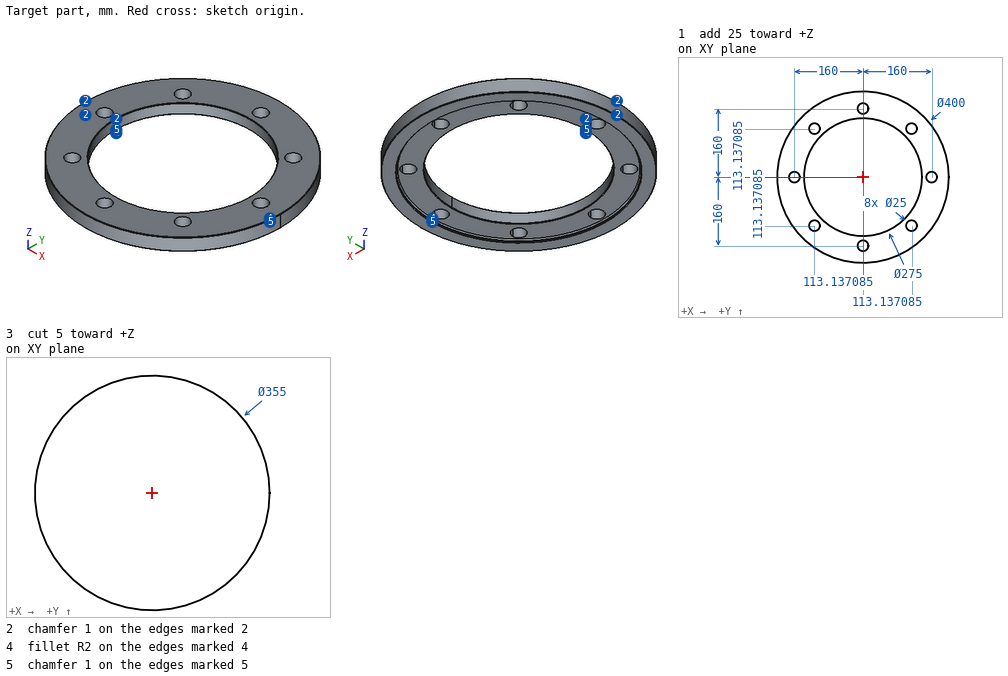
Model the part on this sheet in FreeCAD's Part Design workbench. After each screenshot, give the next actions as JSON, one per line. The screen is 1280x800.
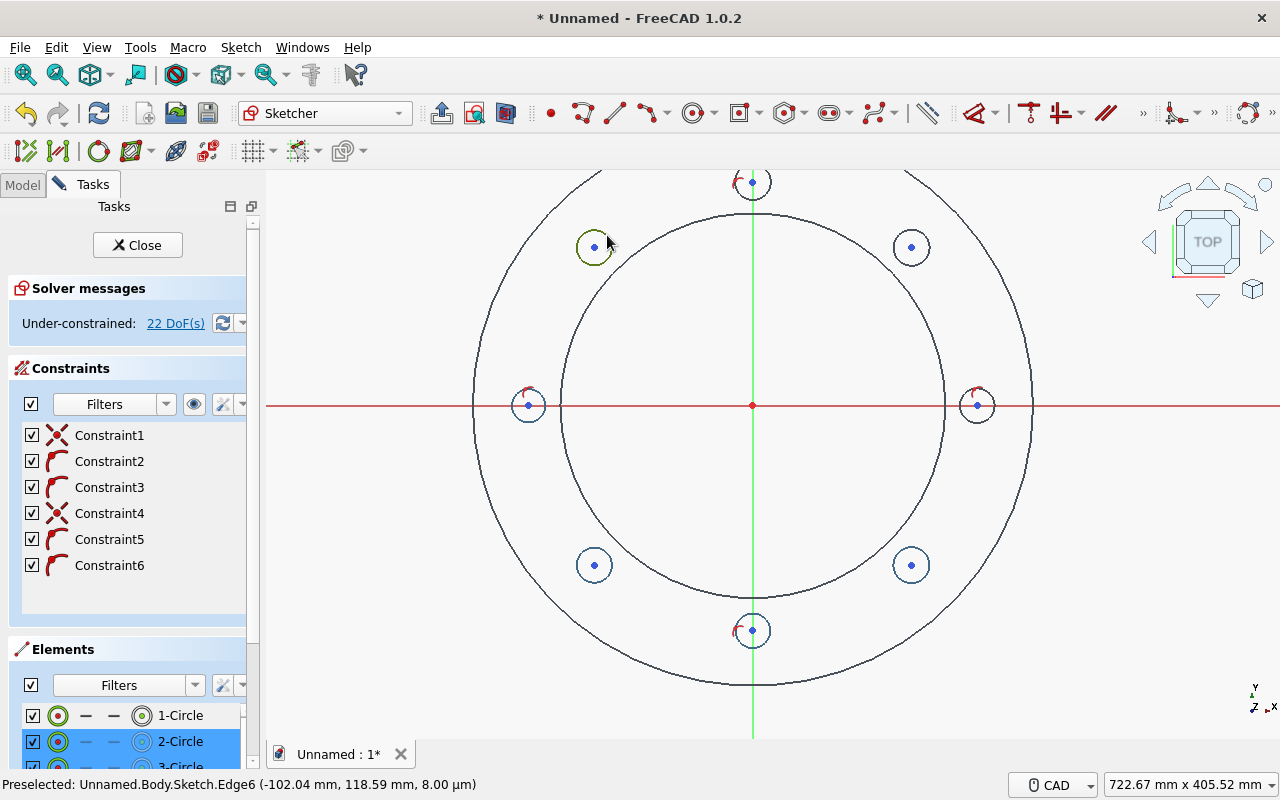
{"action": "left_click", "coordinate": [989, 393]}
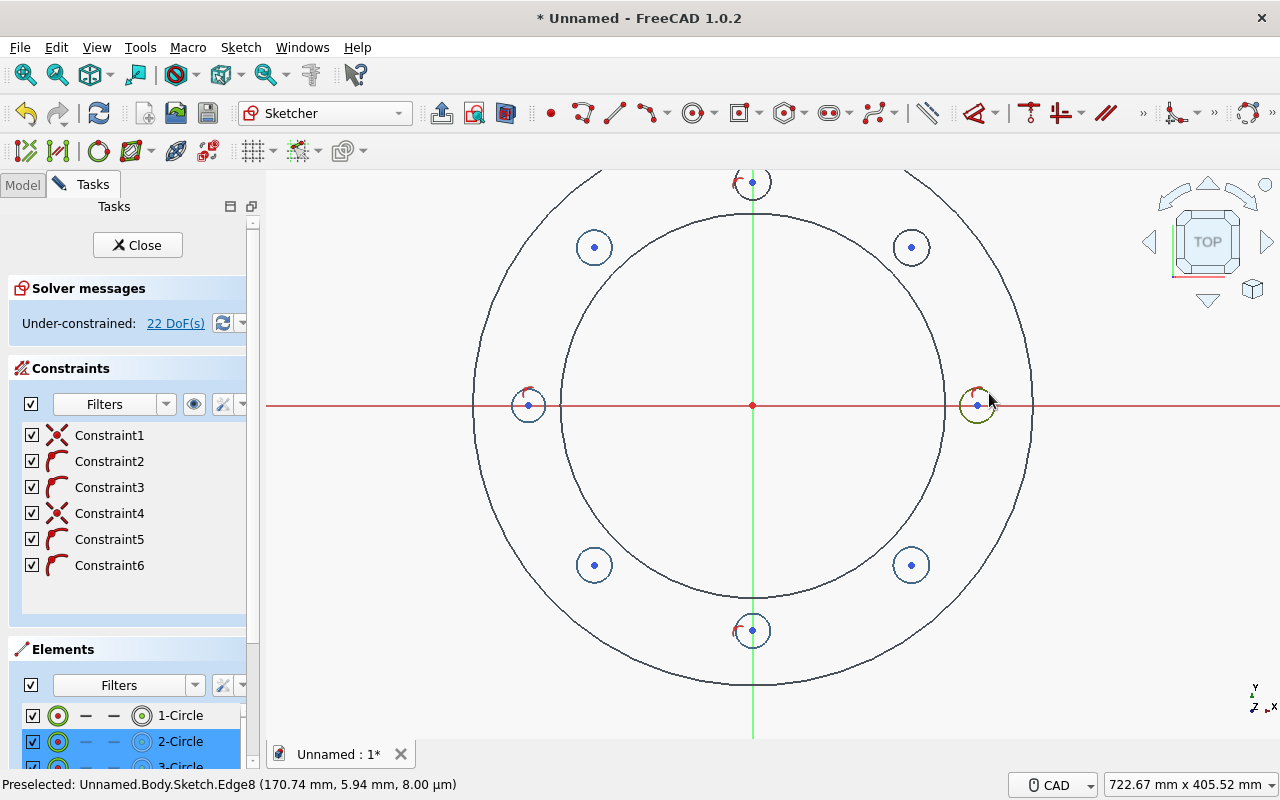
{"action": "left_click", "coordinate": [752, 200]}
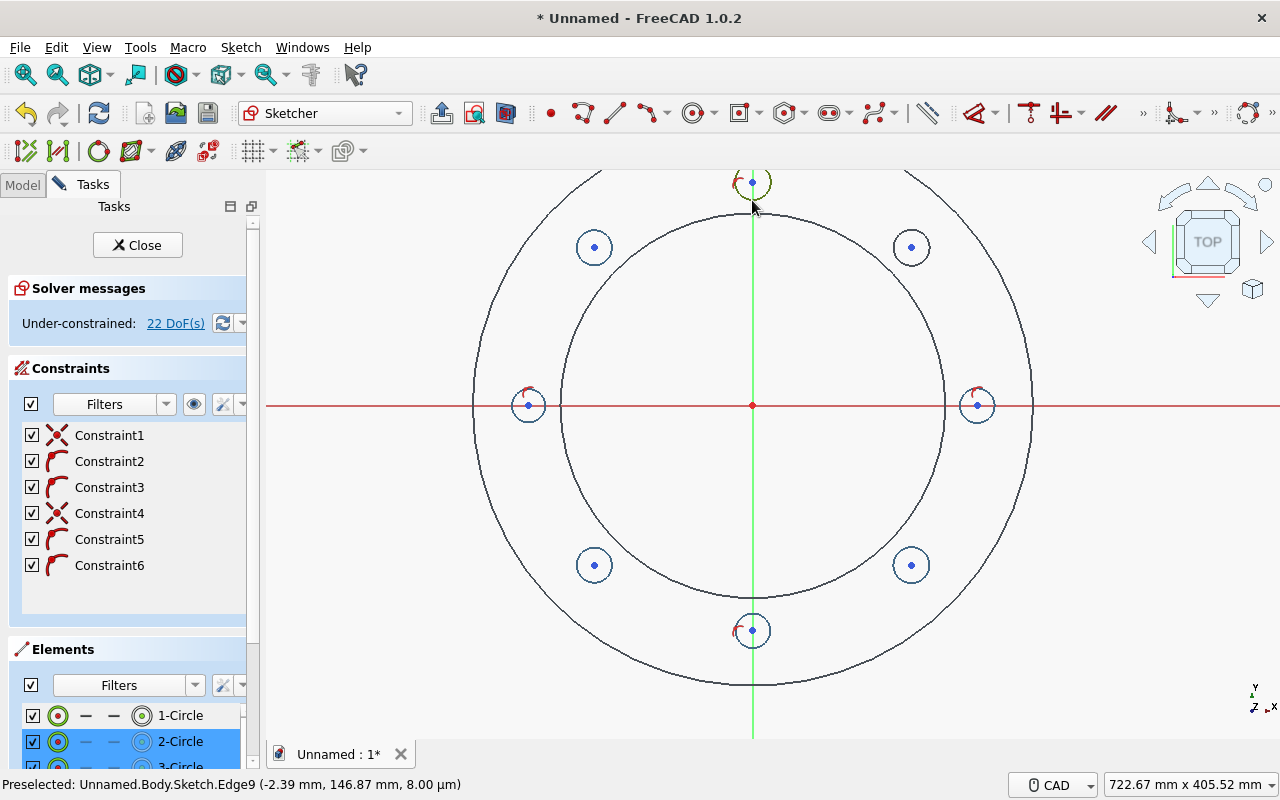
{"action": "left_click", "coordinate": [924, 235]}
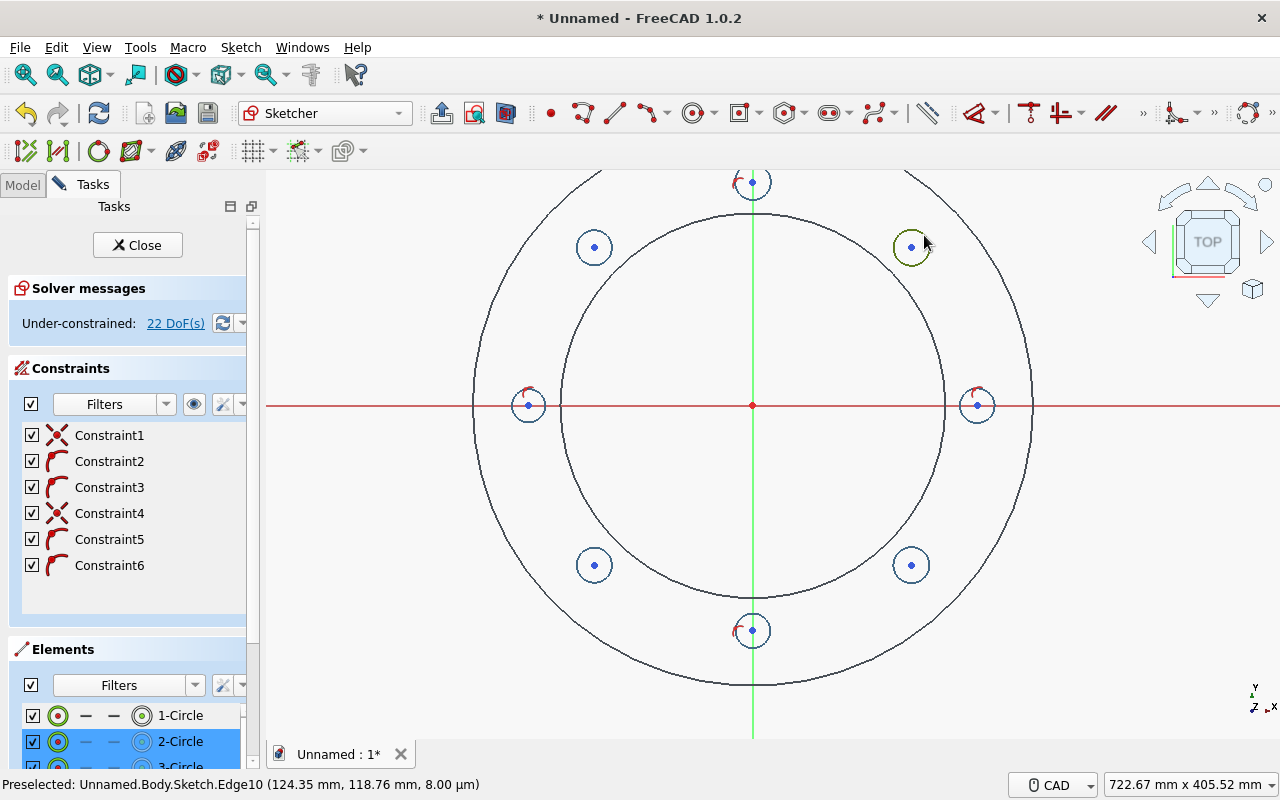
{"action": "key", "text": "e"}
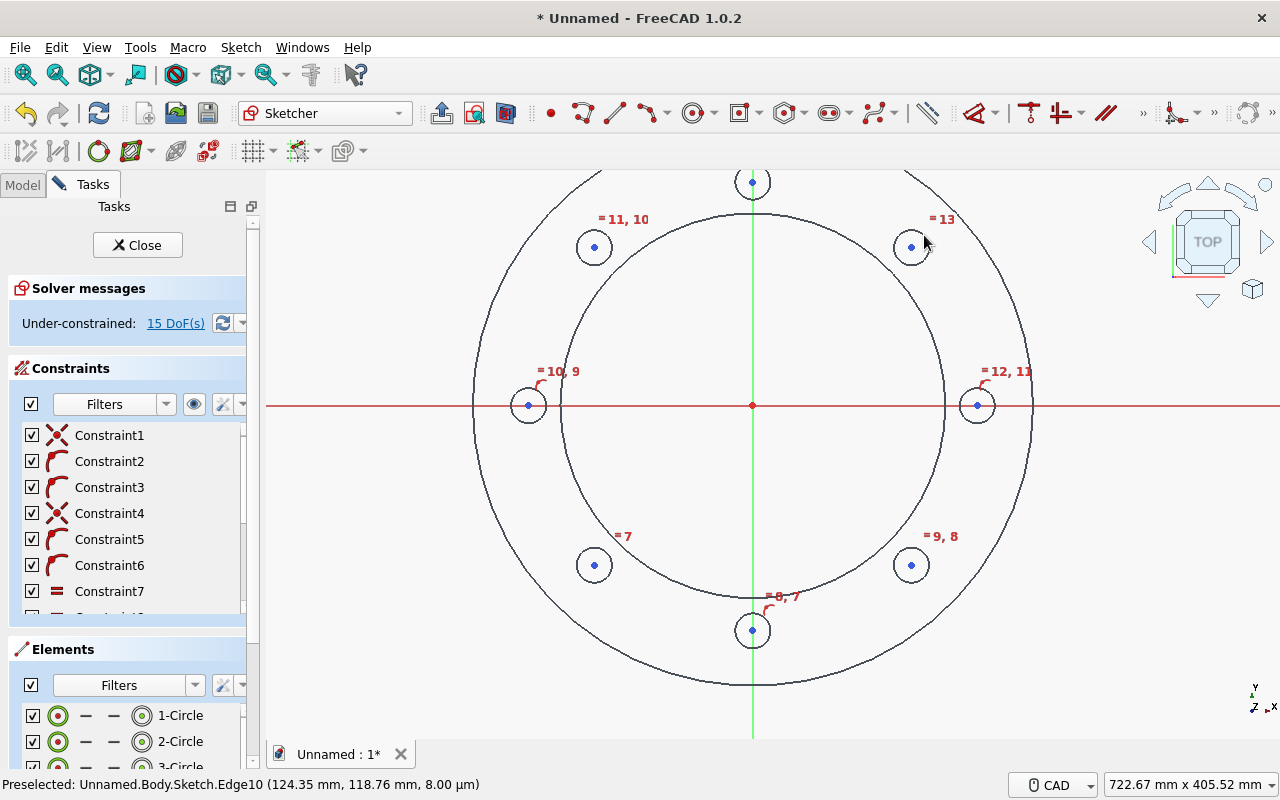
{"action": "left_click", "coordinate": [594, 565]}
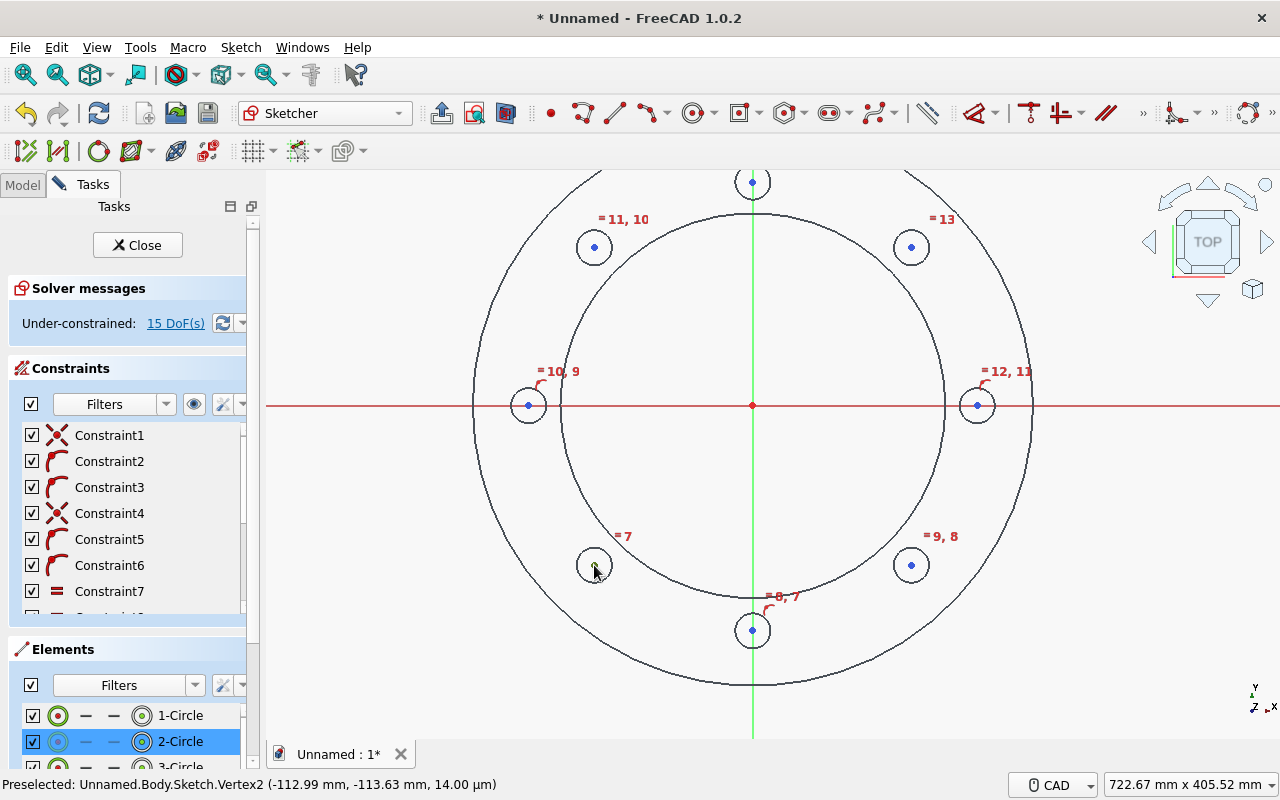
{"action": "left_click", "coordinate": [911, 565]}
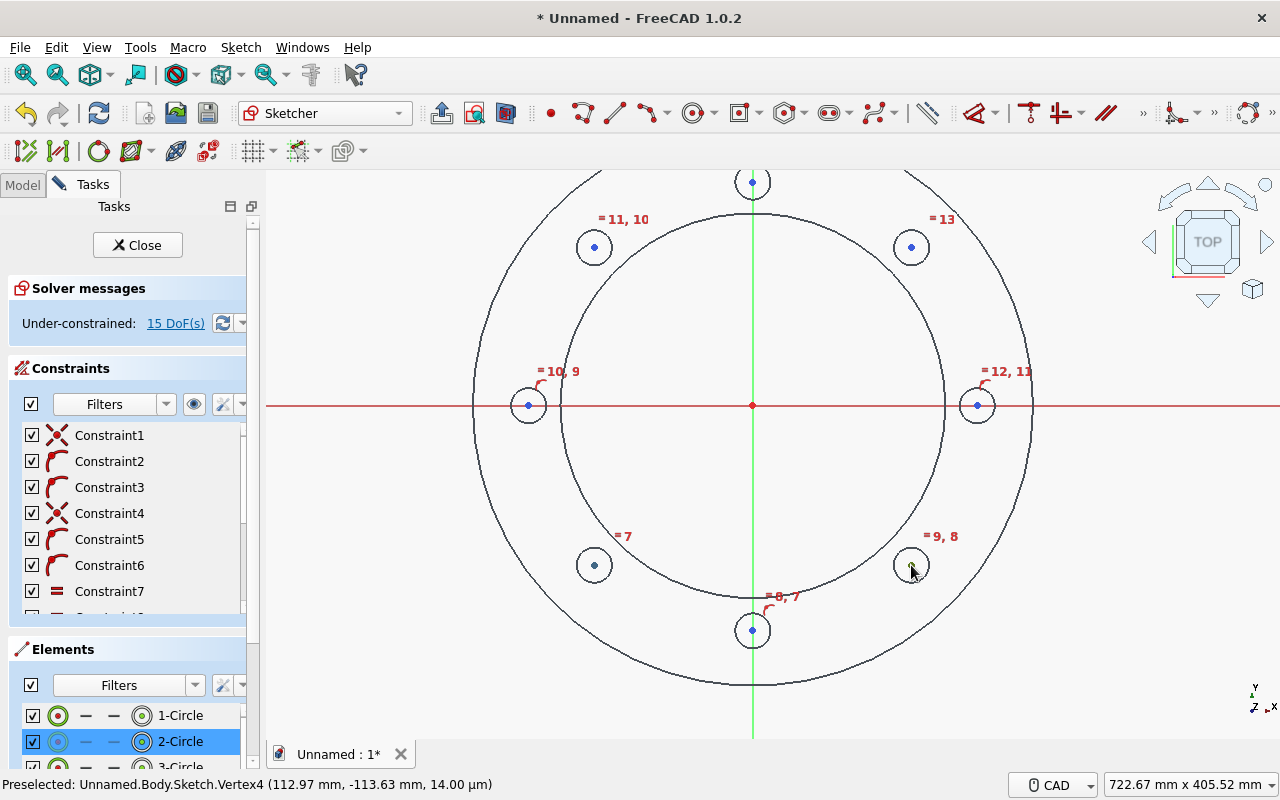
{"action": "left_click", "coordinate": [1084, 114]}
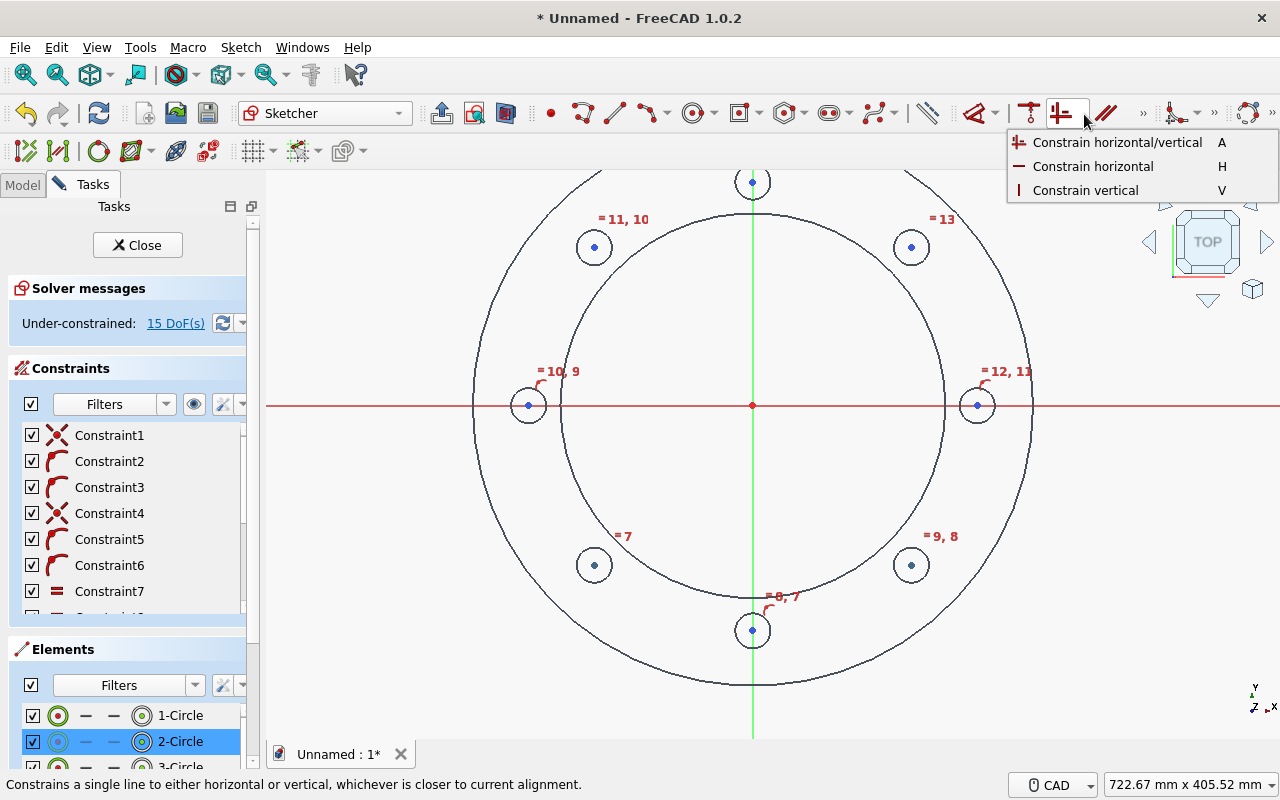
{"action": "left_click", "coordinate": [1143, 166]}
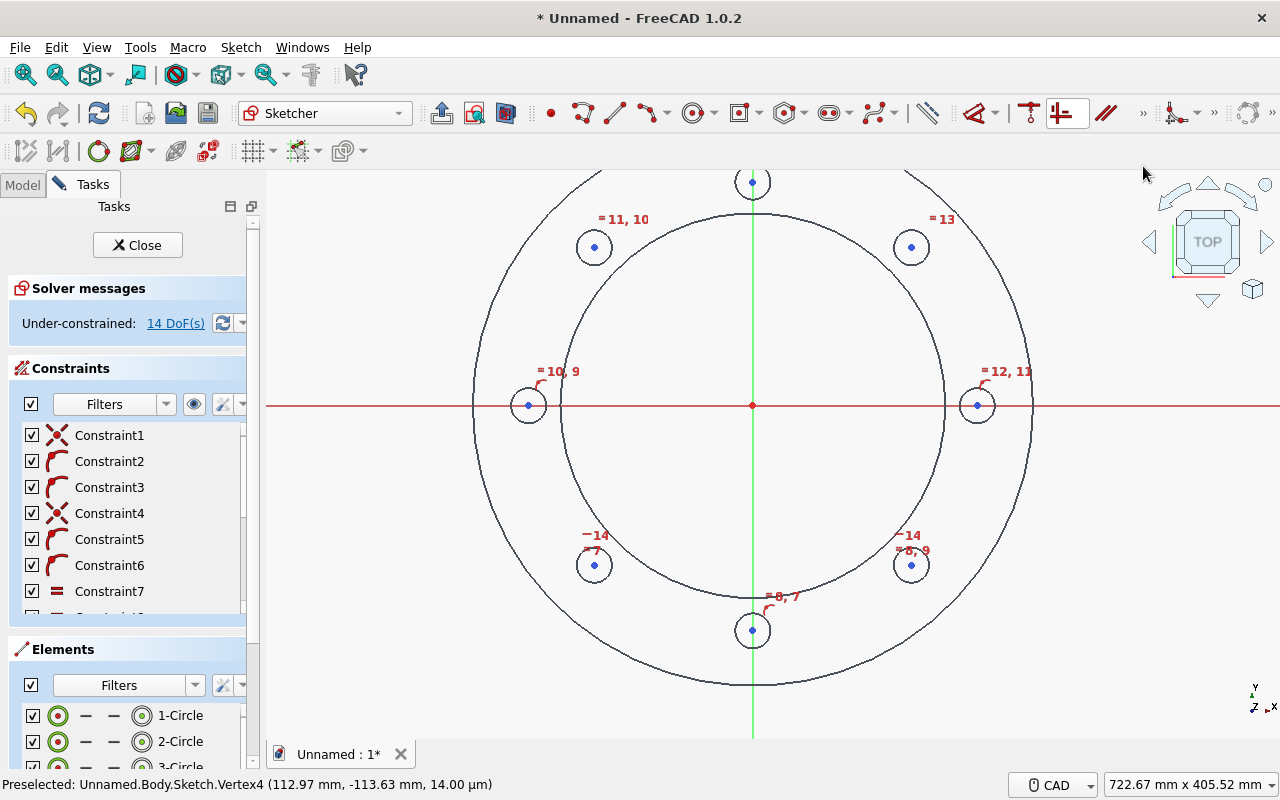
{"action": "left_click", "coordinate": [594, 565]}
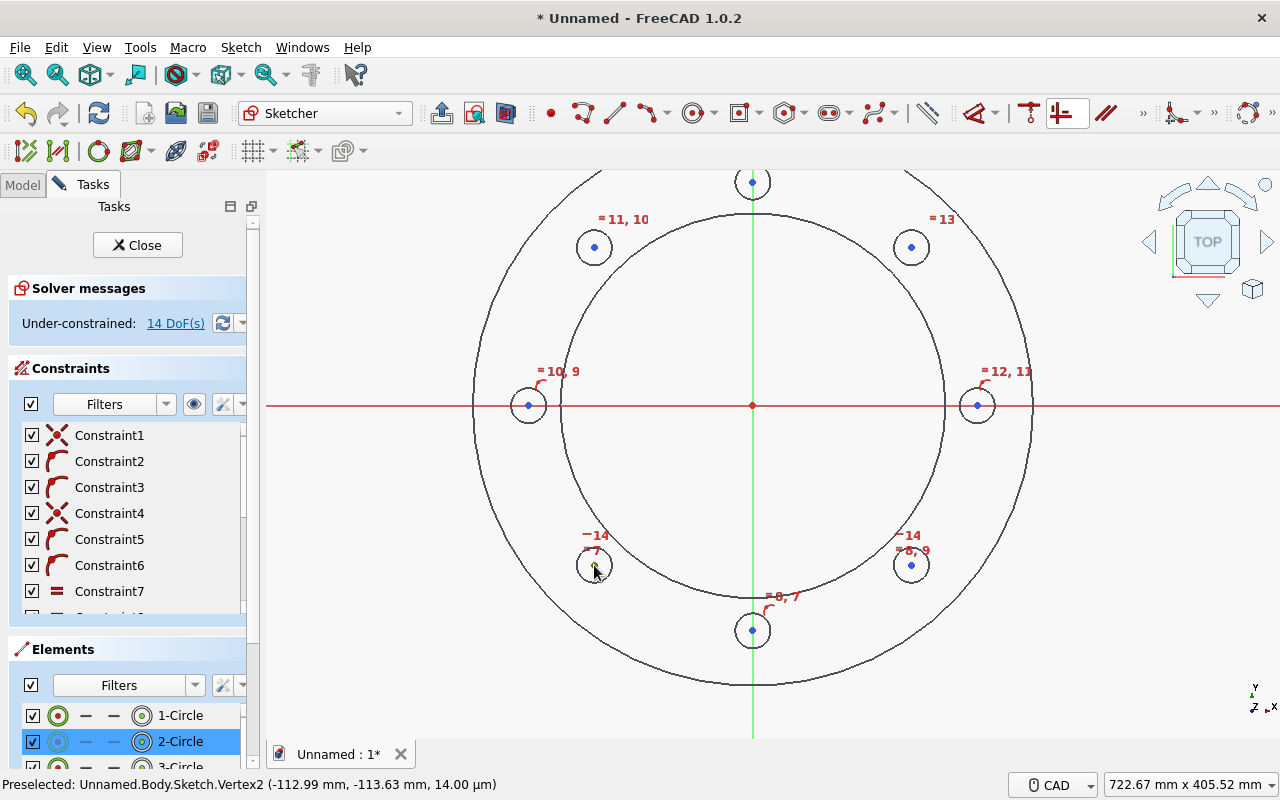
{"action": "left_click", "coordinate": [594, 248]}